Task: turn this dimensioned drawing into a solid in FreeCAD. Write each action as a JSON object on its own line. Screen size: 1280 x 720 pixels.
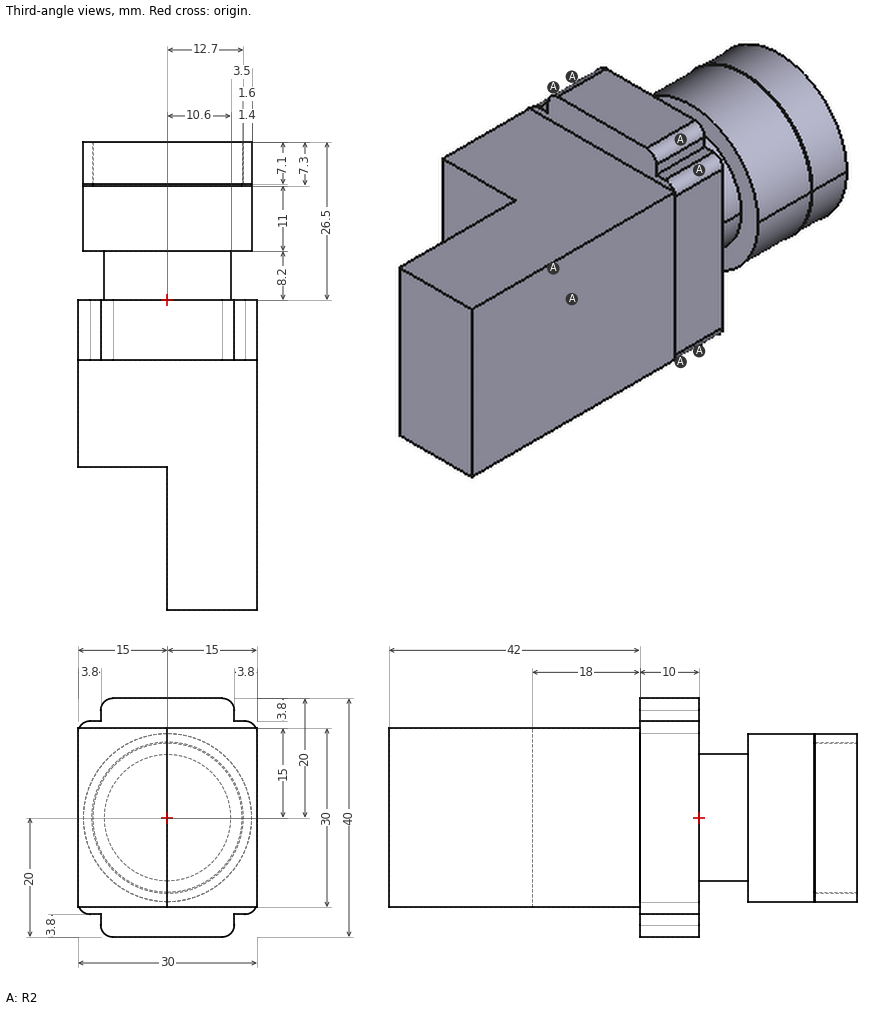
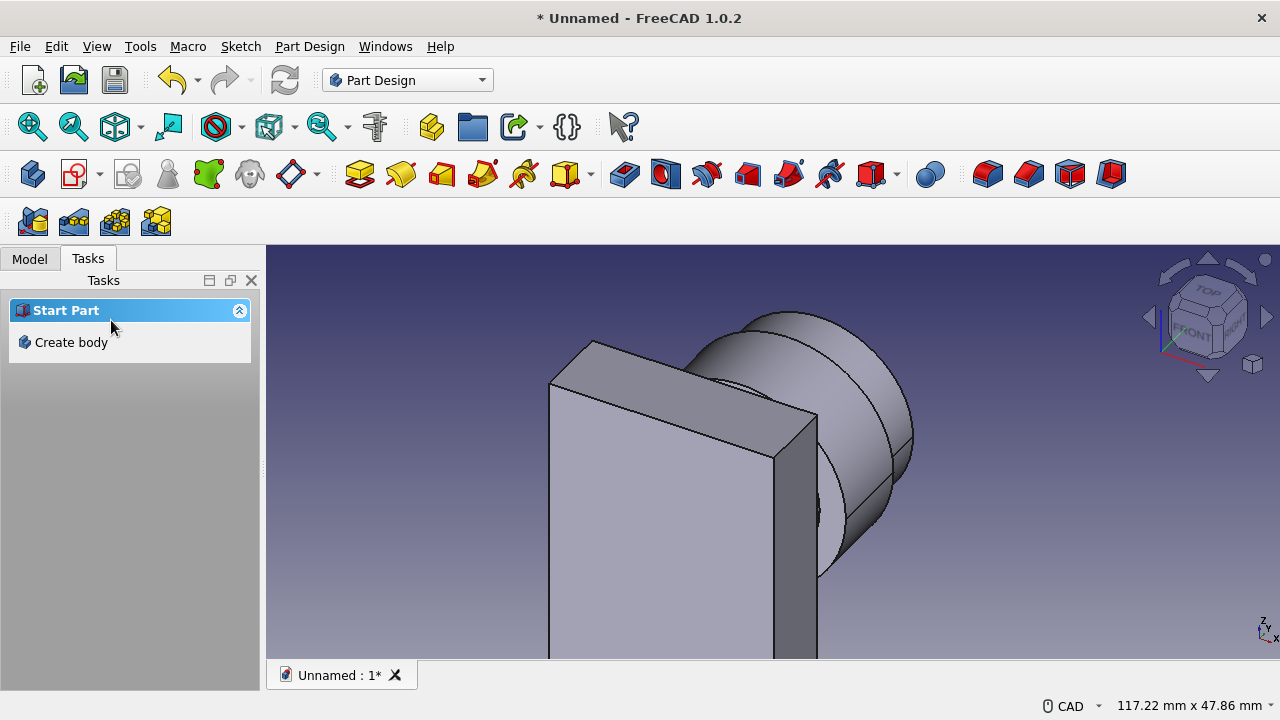
{"action": "left_click", "coordinate": [33, 128]}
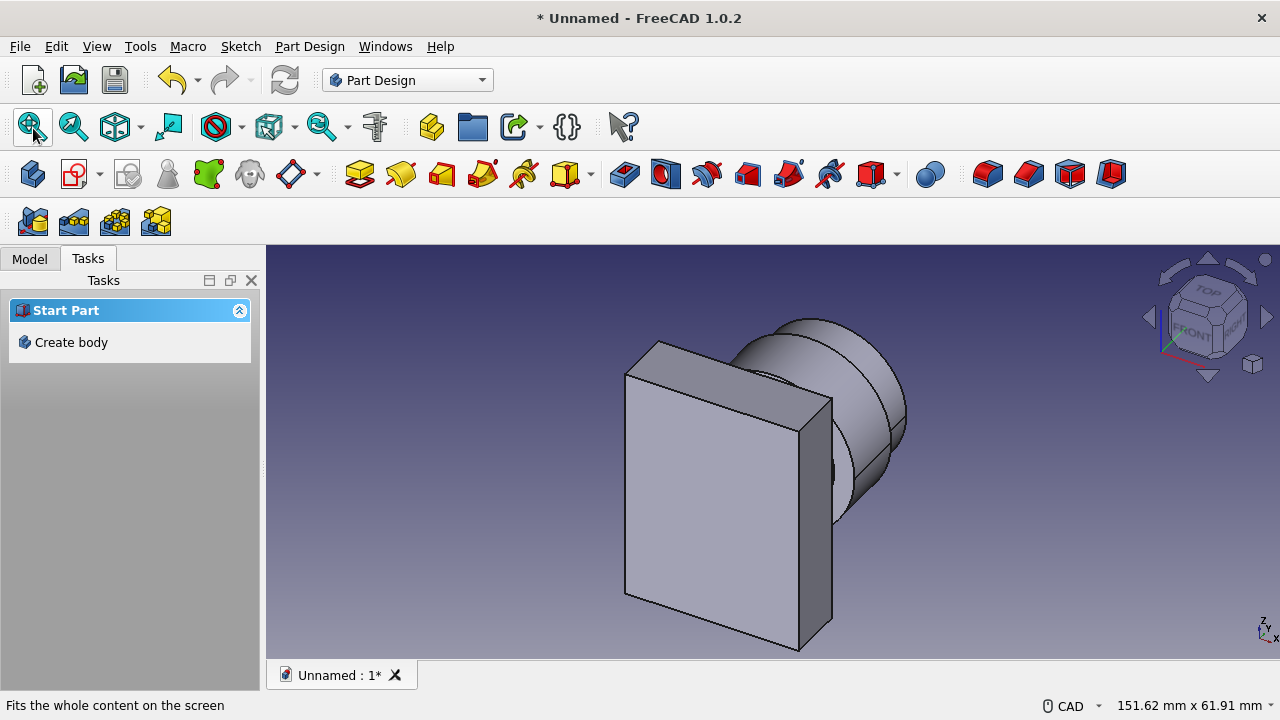
{"action": "left_click", "coordinate": [74, 174]}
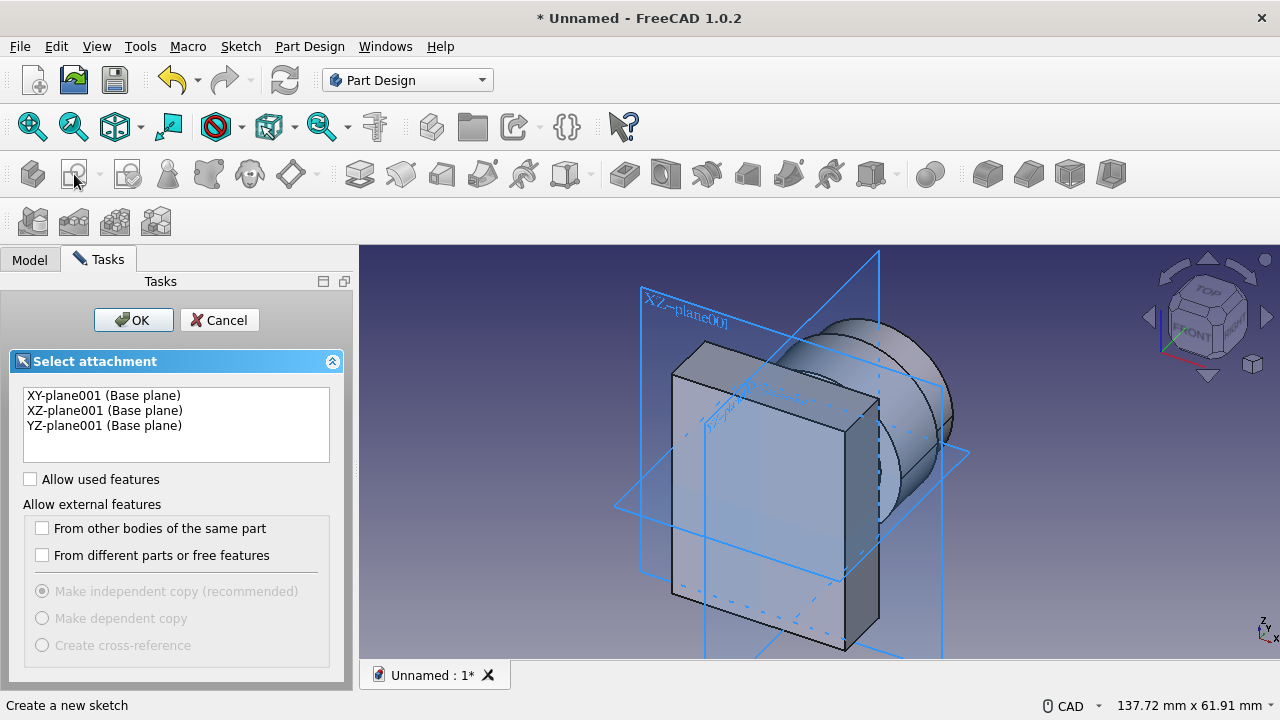
{"action": "left_click", "coordinate": [84, 410]}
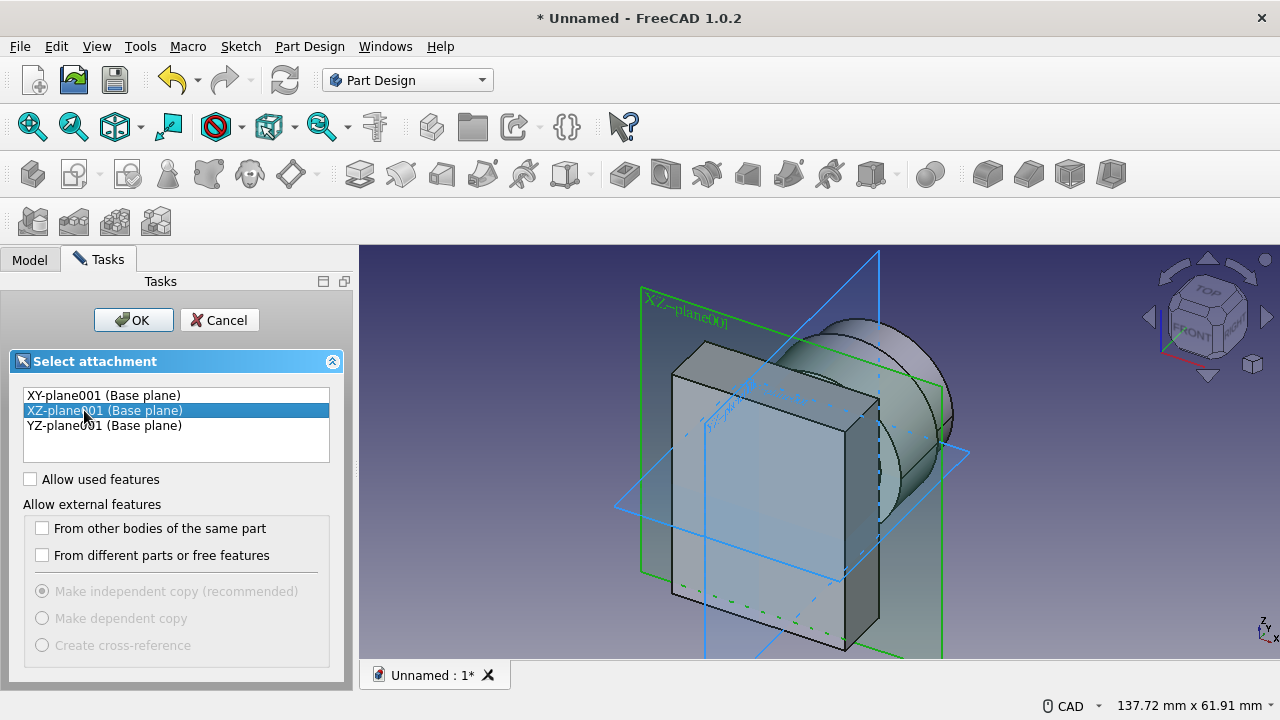
{"action": "left_click", "coordinate": [134, 320]}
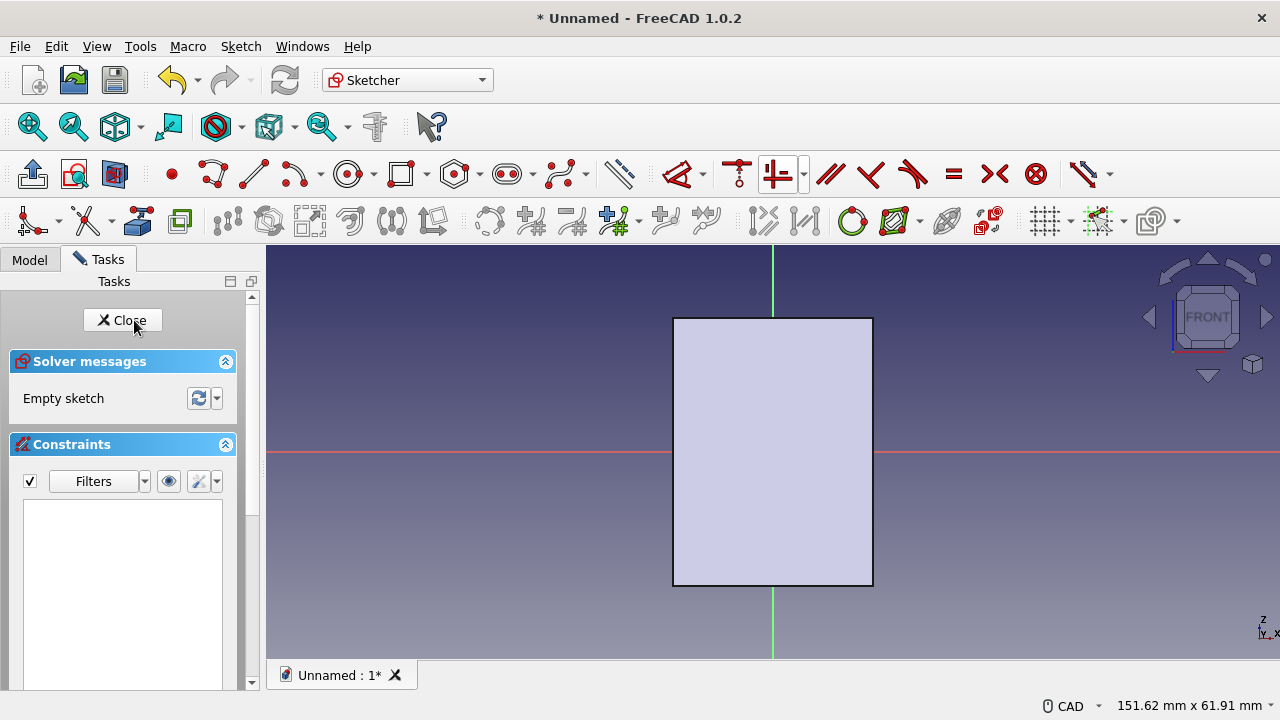
{"action": "left_click", "coordinate": [115, 174]}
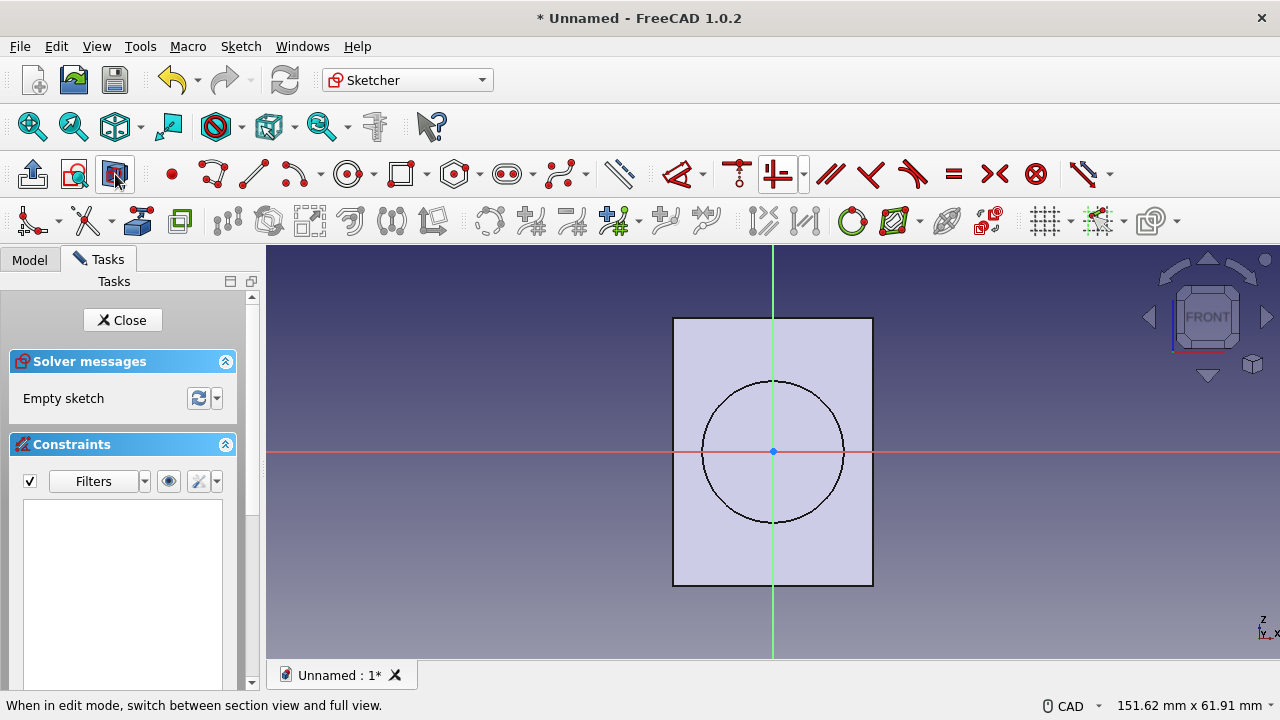
{"action": "key", "text": "g r"}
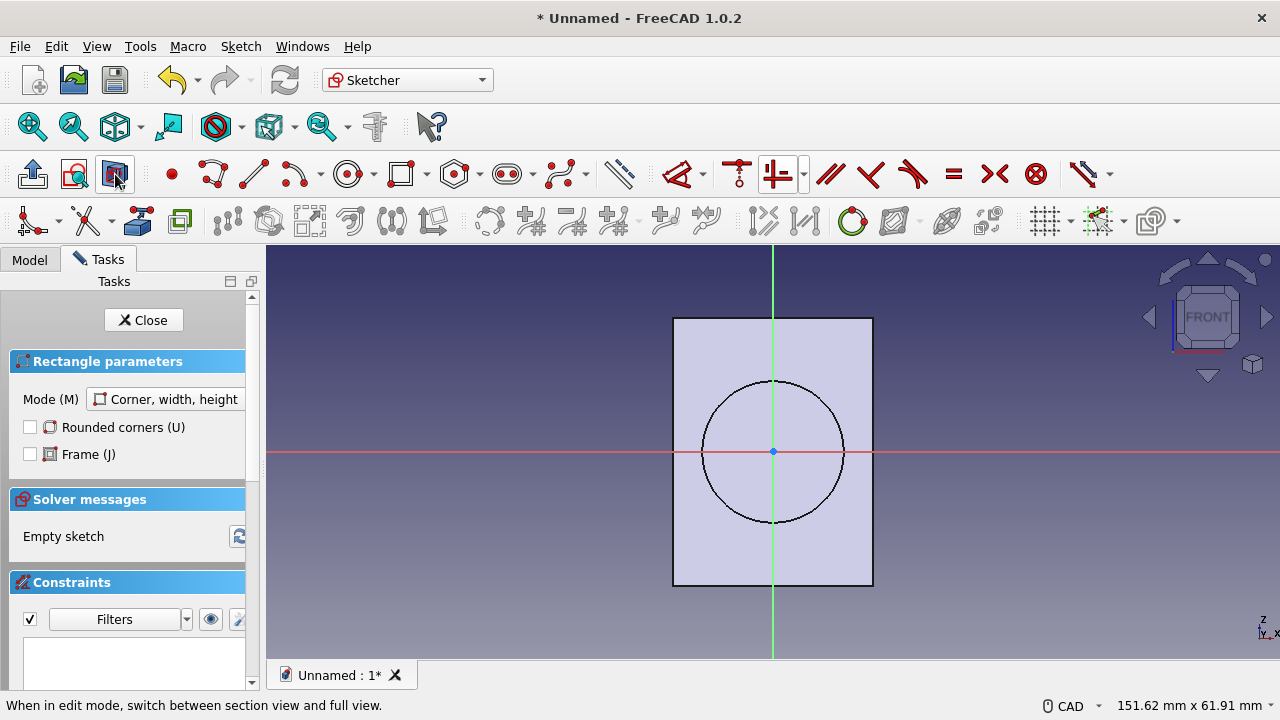
{"action": "left_click", "coordinate": [848, 318]}
{"action": "mouse_move", "coordinate": [873, 344]}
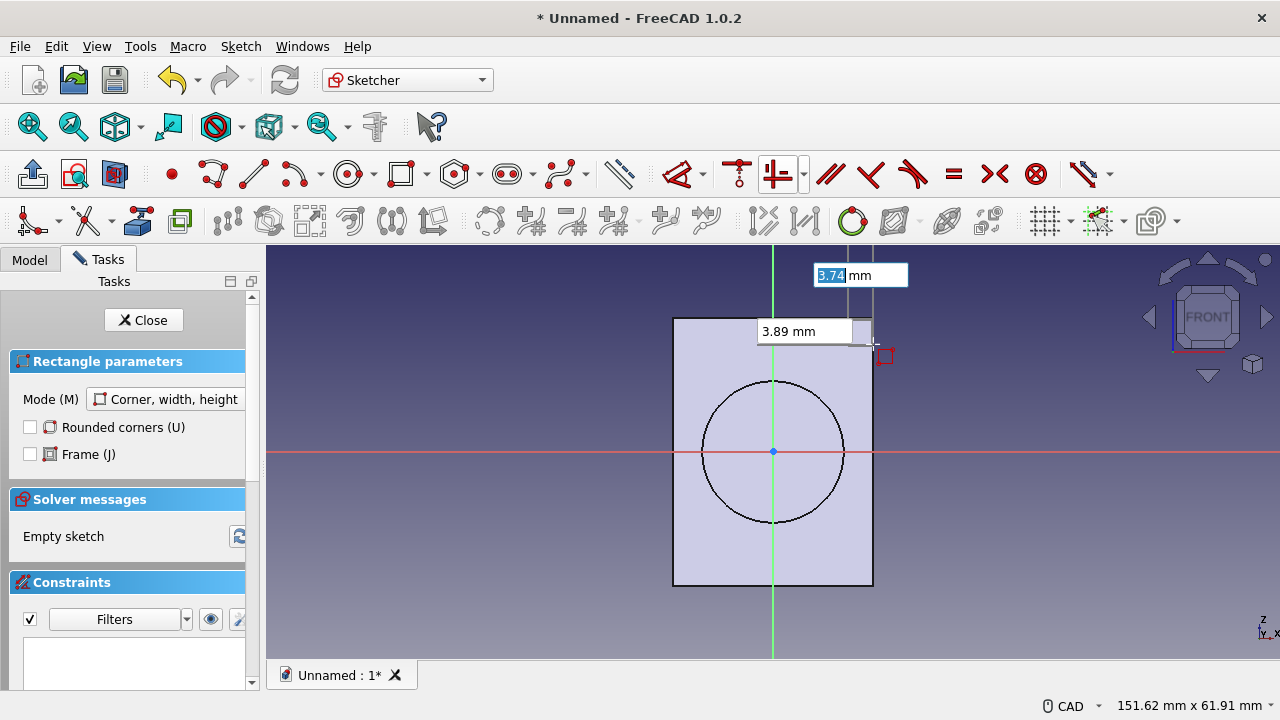
{"action": "type", "text": "3.8"}
{"action": "key", "text": "Tab"}
{"action": "type", "text": "3.8"}
{"action": "key", "text": "Return"}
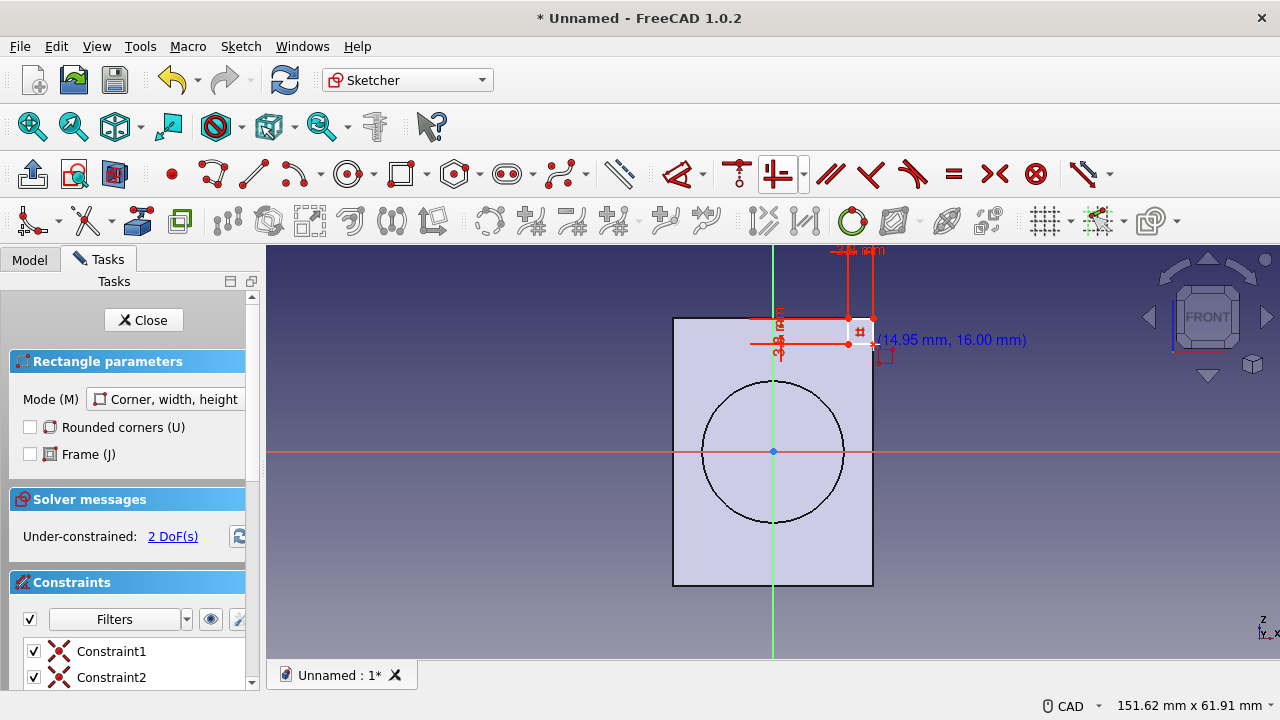
{"action": "left_click", "coordinate": [673, 318]}
{"action": "mouse_move", "coordinate": [698, 344]}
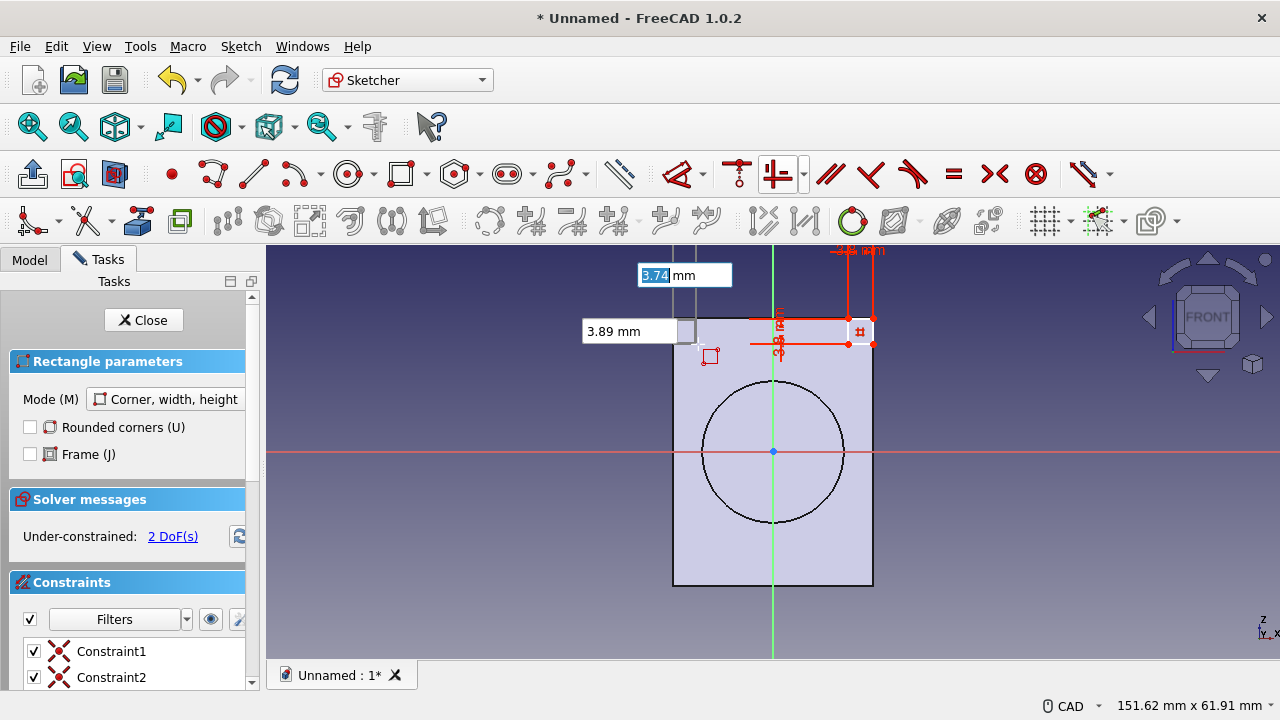
{"action": "type", "text": "3.8"}
{"action": "key", "text": "Tab"}
{"action": "type", "text": "3.8"}
{"action": "key", "text": "Return"}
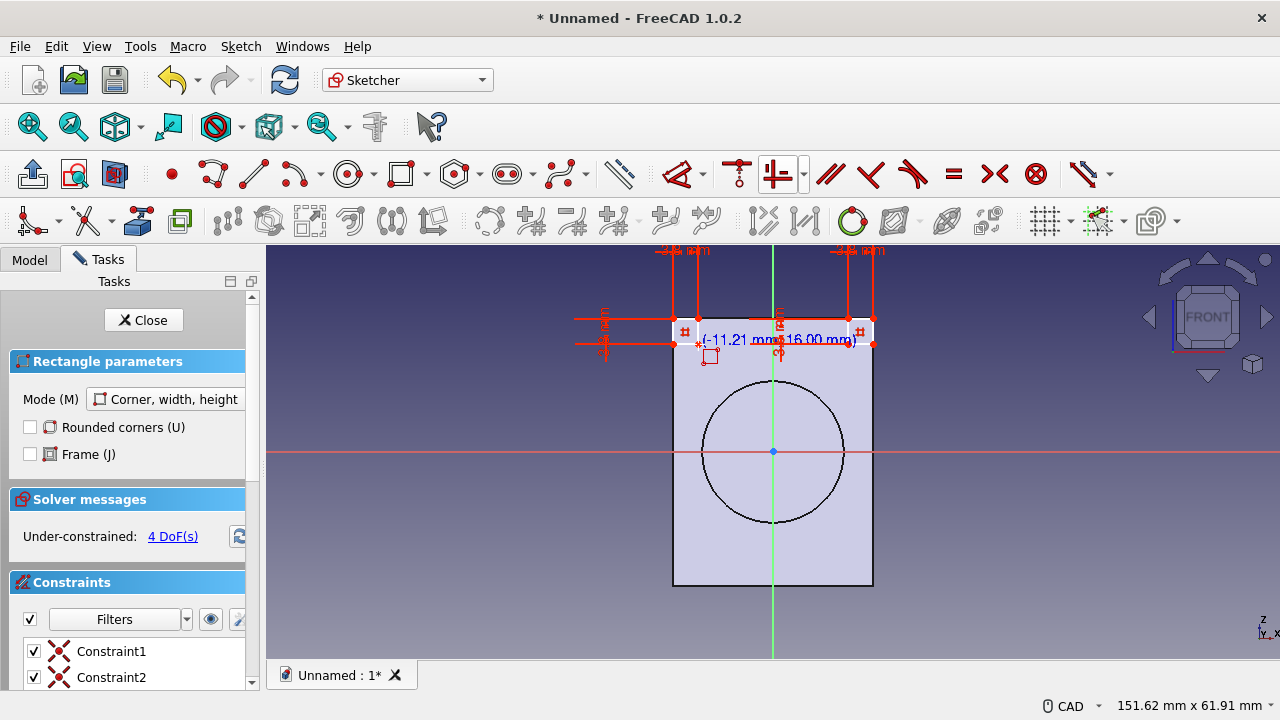
{"action": "left_click", "coordinate": [673, 560]}
{"action": "mouse_move", "coordinate": [698, 586]}